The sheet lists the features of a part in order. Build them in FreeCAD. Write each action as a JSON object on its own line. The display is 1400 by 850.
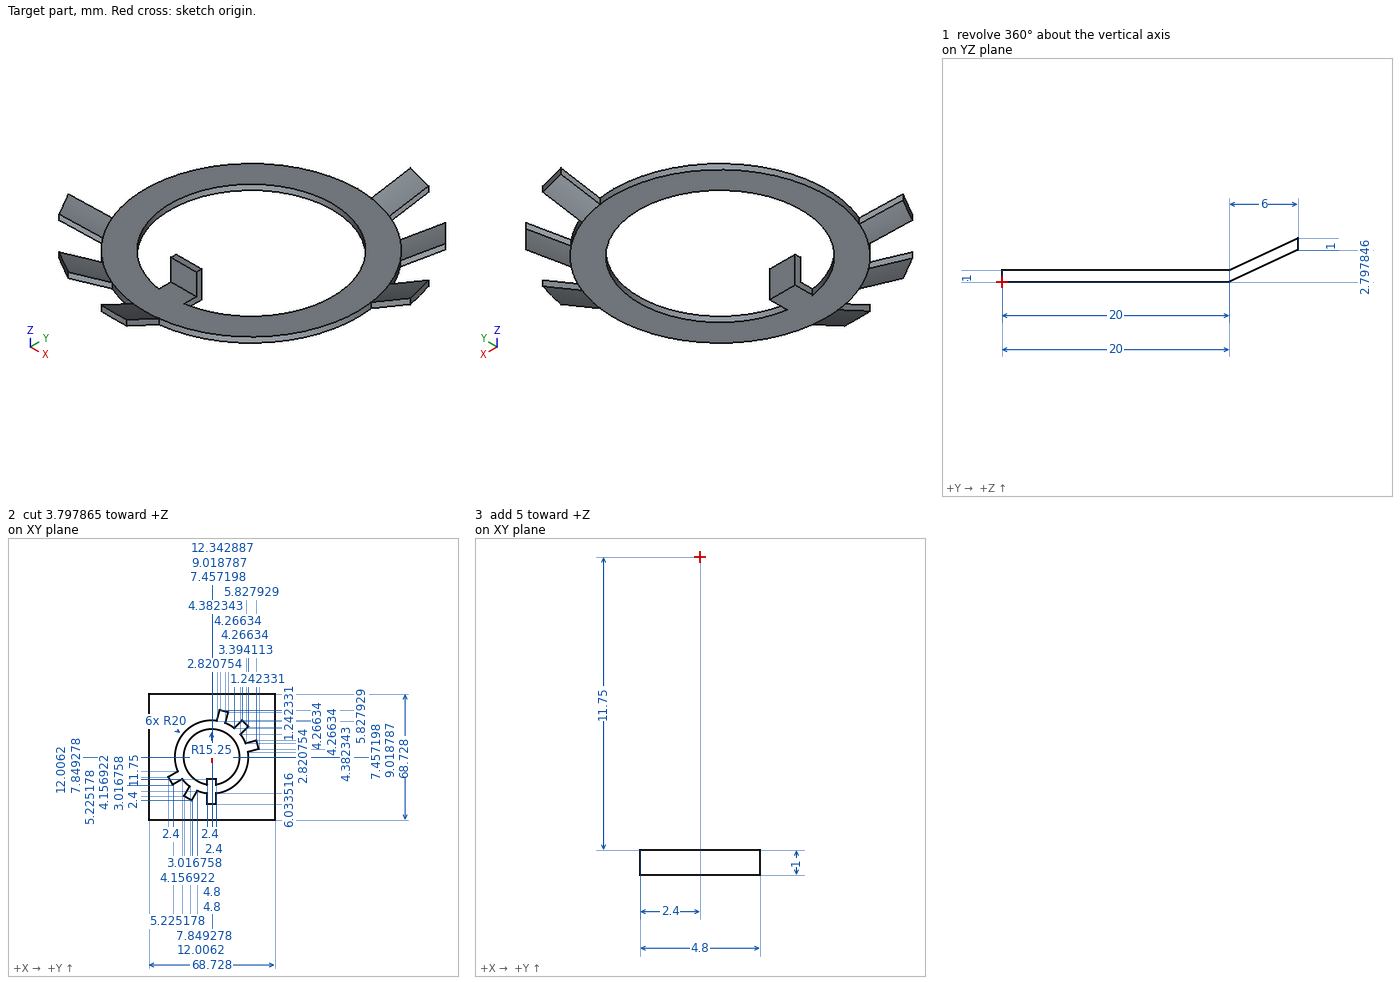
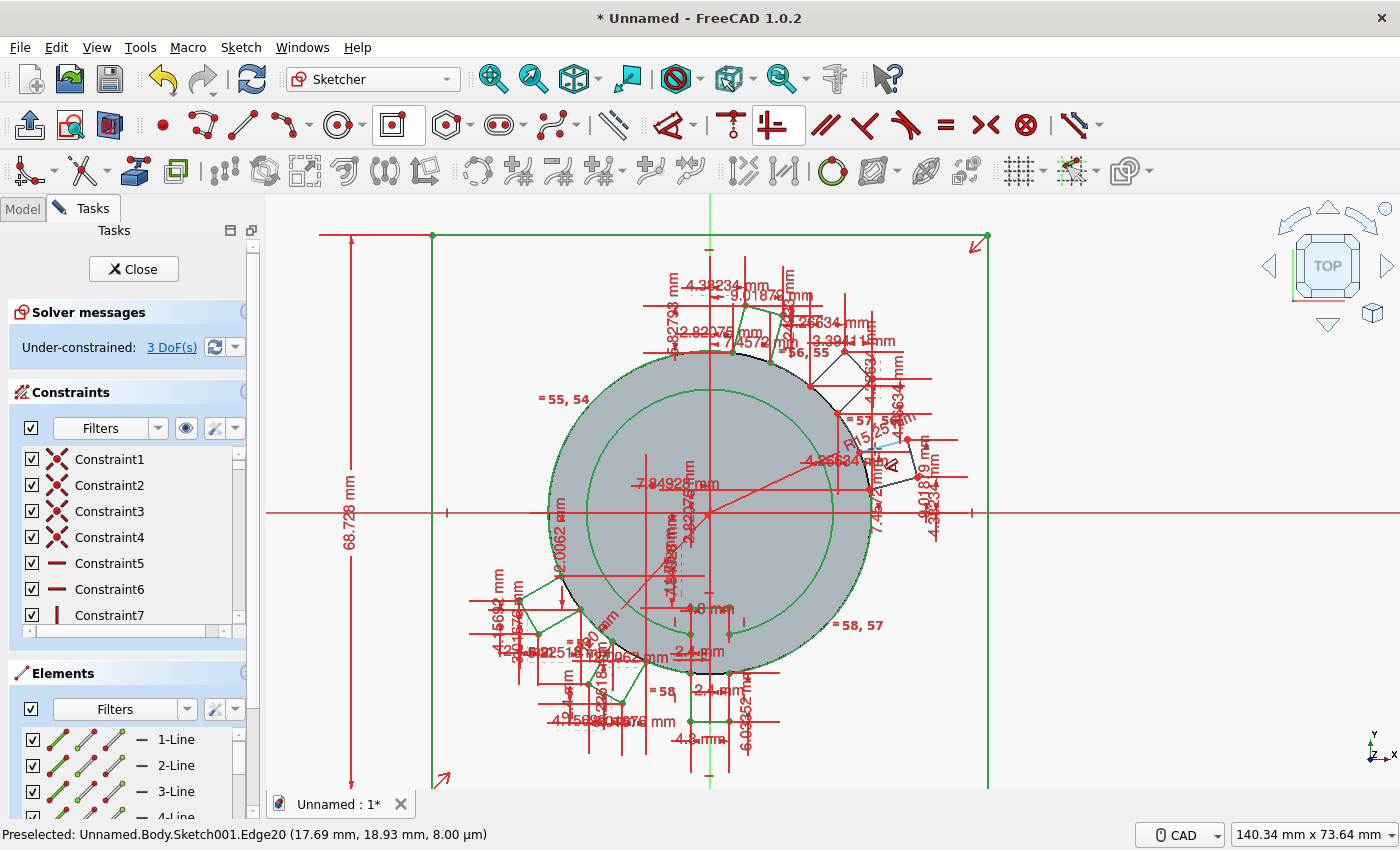
{"action": "left_click", "coordinate": [874, 449]}
{"action": "left_click", "coordinate": [884, 534]}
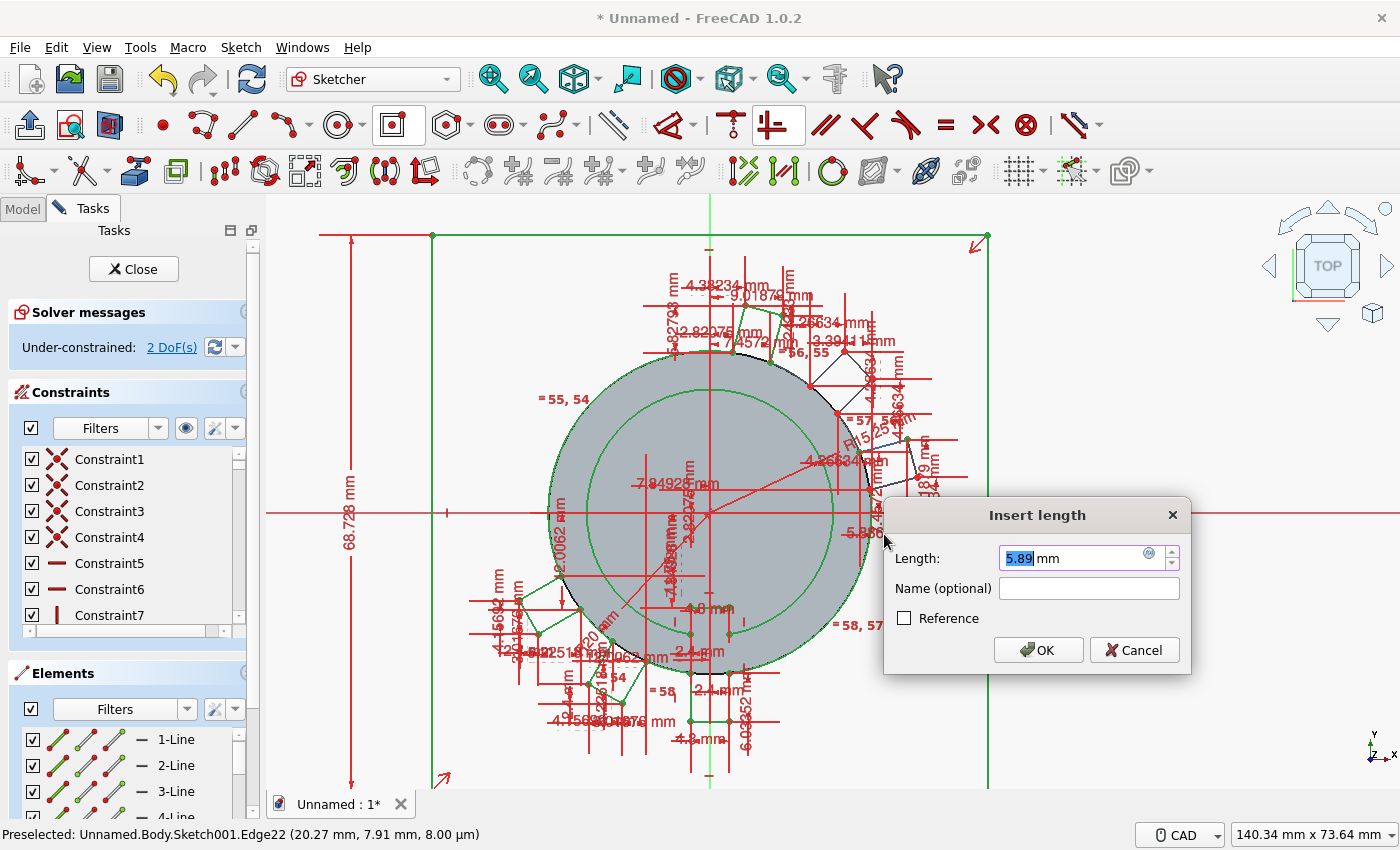
{"action": "type", "text": "5.827929"}
{"action": "key", "text": "Return"}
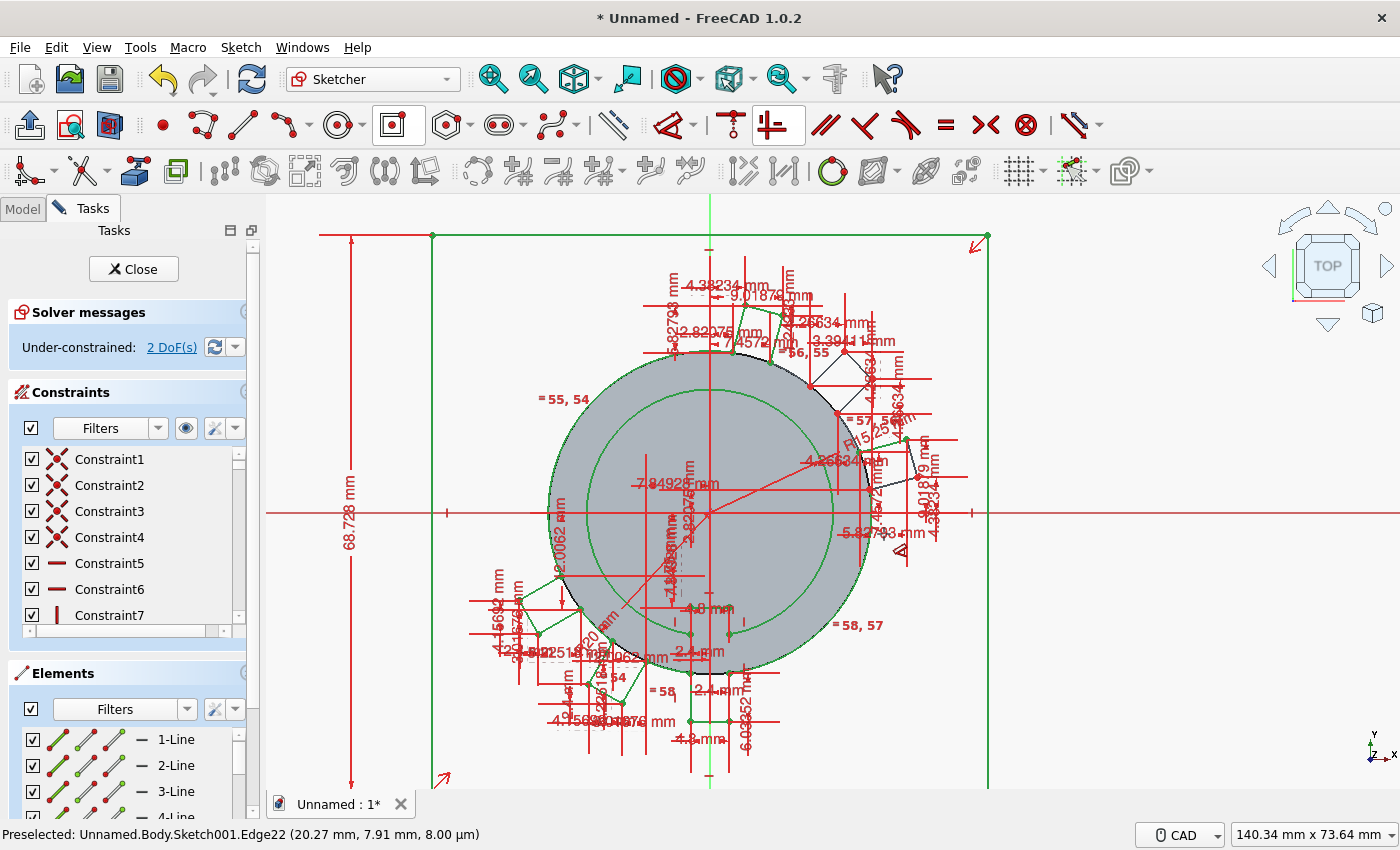
{"action": "scroll", "coordinate": [910, 451], "scroll_direction": "up", "scroll_amount": 7}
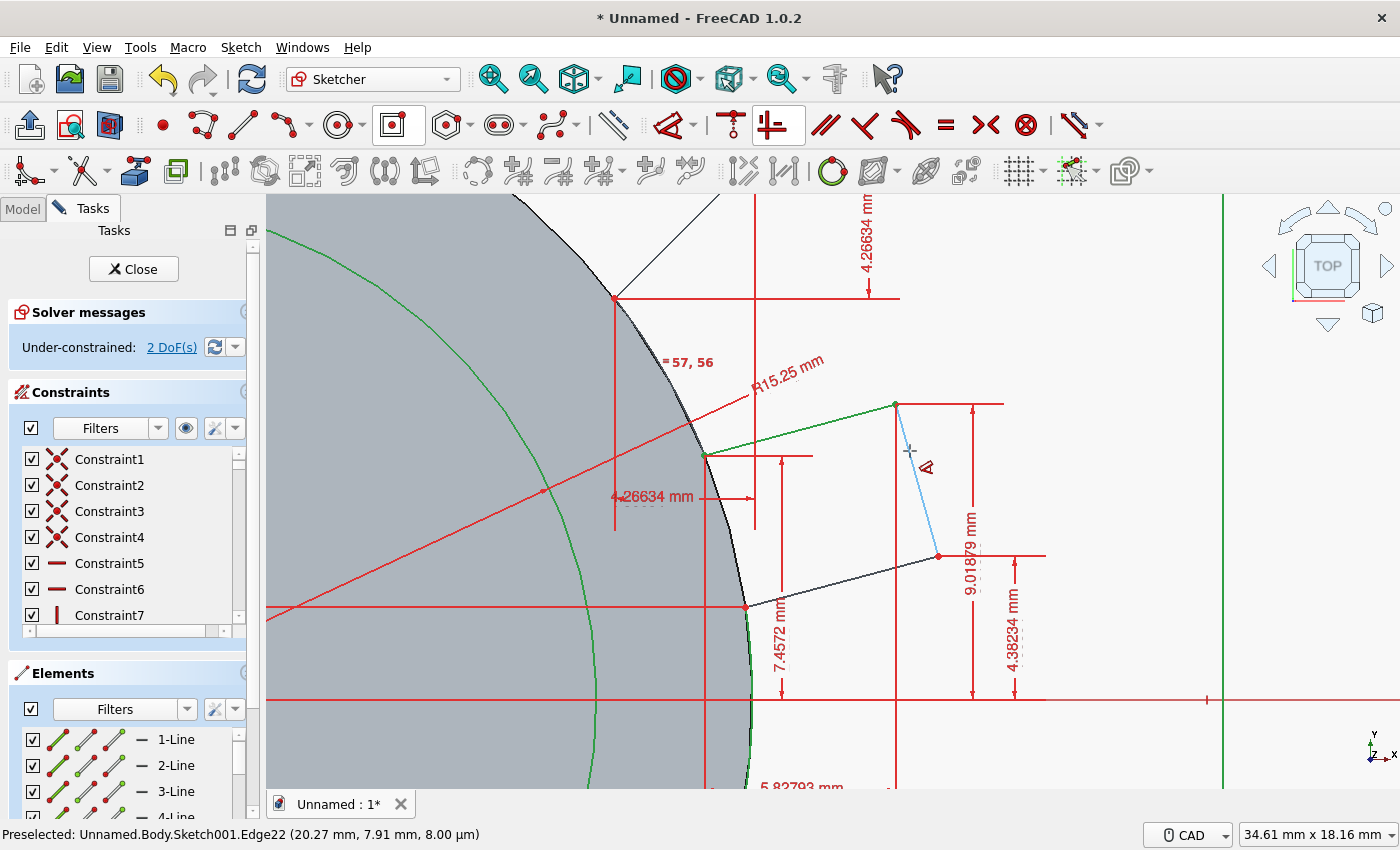
{"action": "left_click", "coordinate": [909, 450]}
{"action": "left_click", "coordinate": [917, 370]}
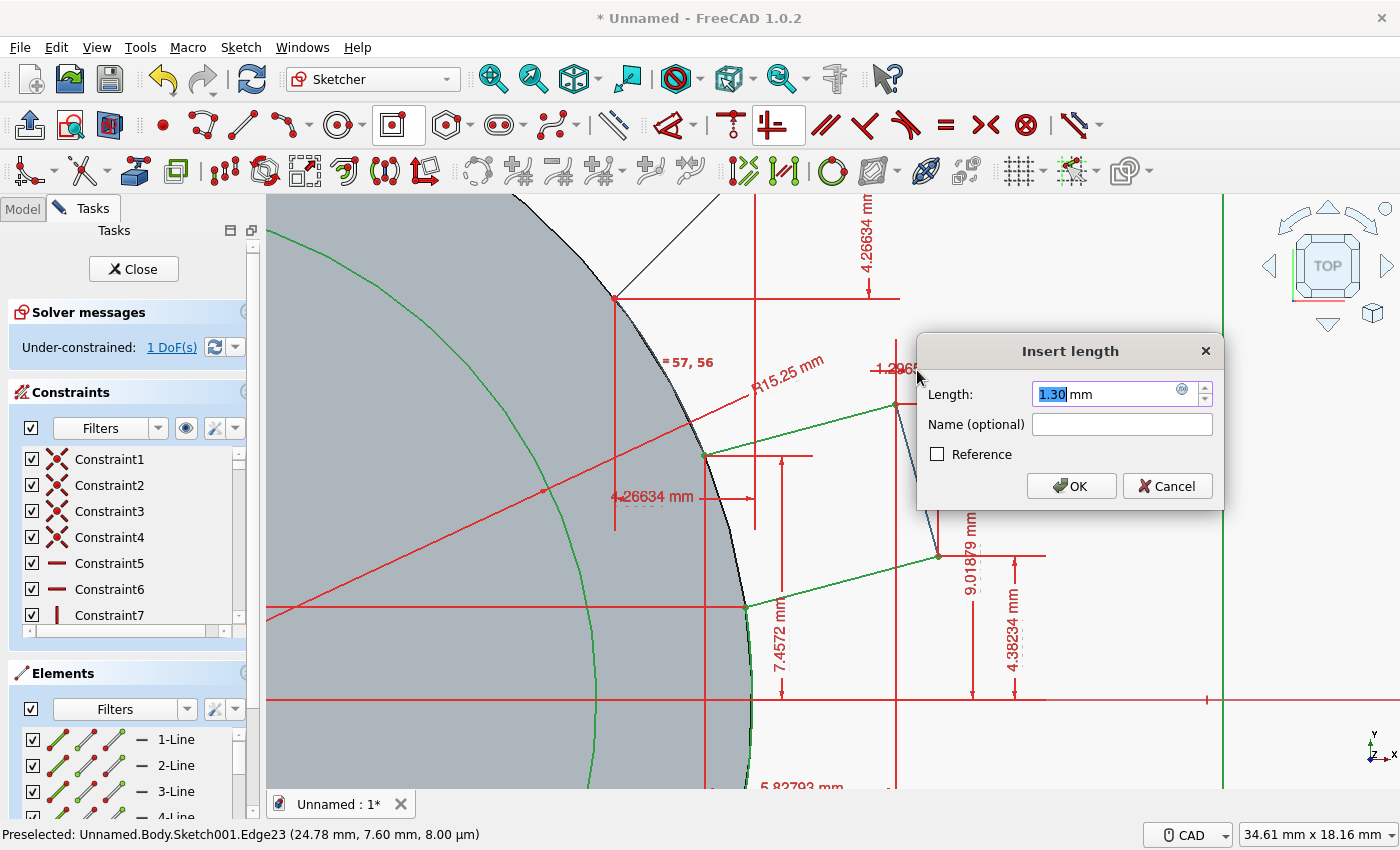
{"action": "type", "text": "1.242331"}
{"action": "key", "text": "Return"}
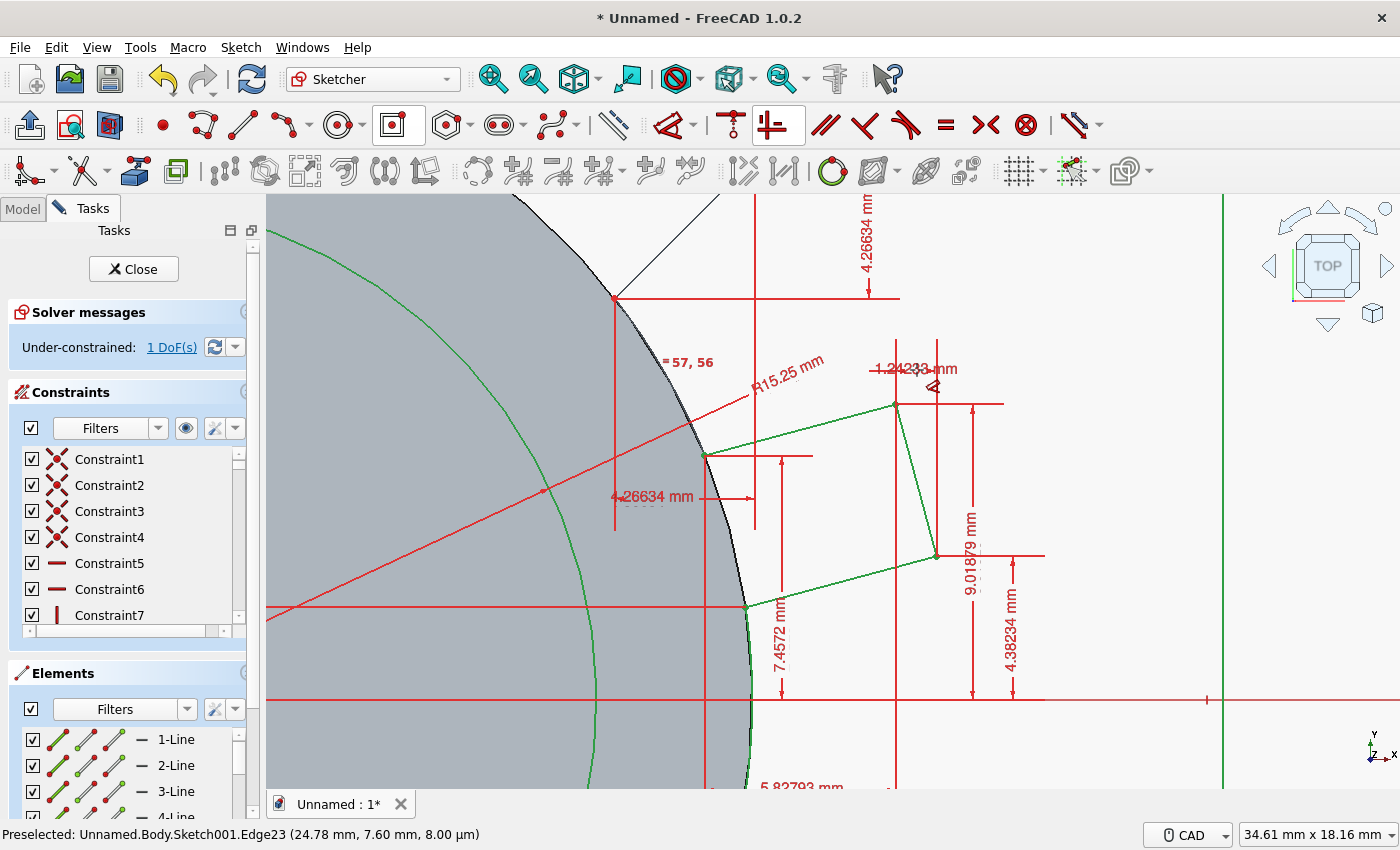
{"action": "scroll", "coordinate": [897, 450], "scroll_direction": "down", "scroll_amount": 9}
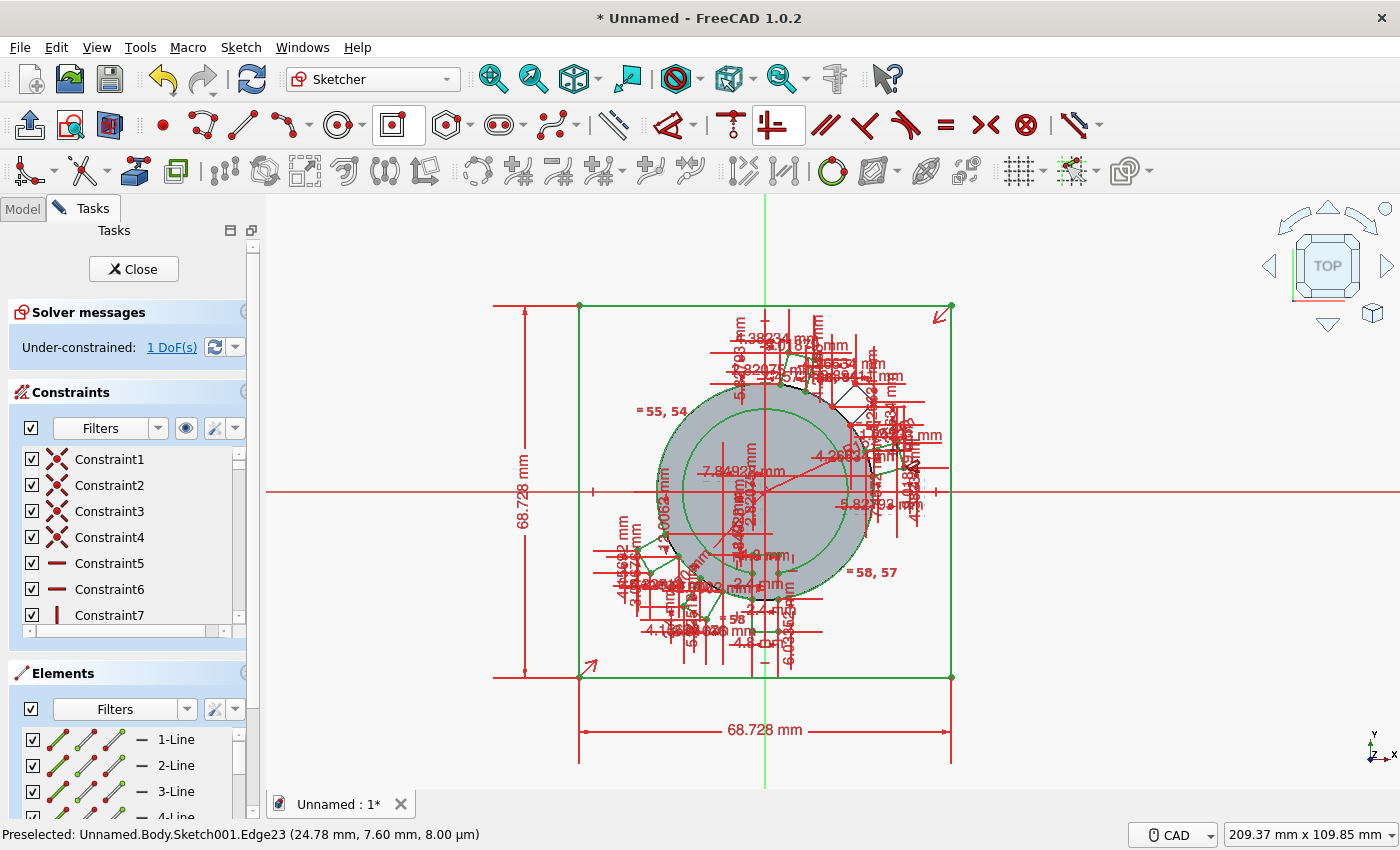
{"action": "left_click", "coordinate": [832, 407]}
{"action": "left_click", "coordinate": [799, 277]}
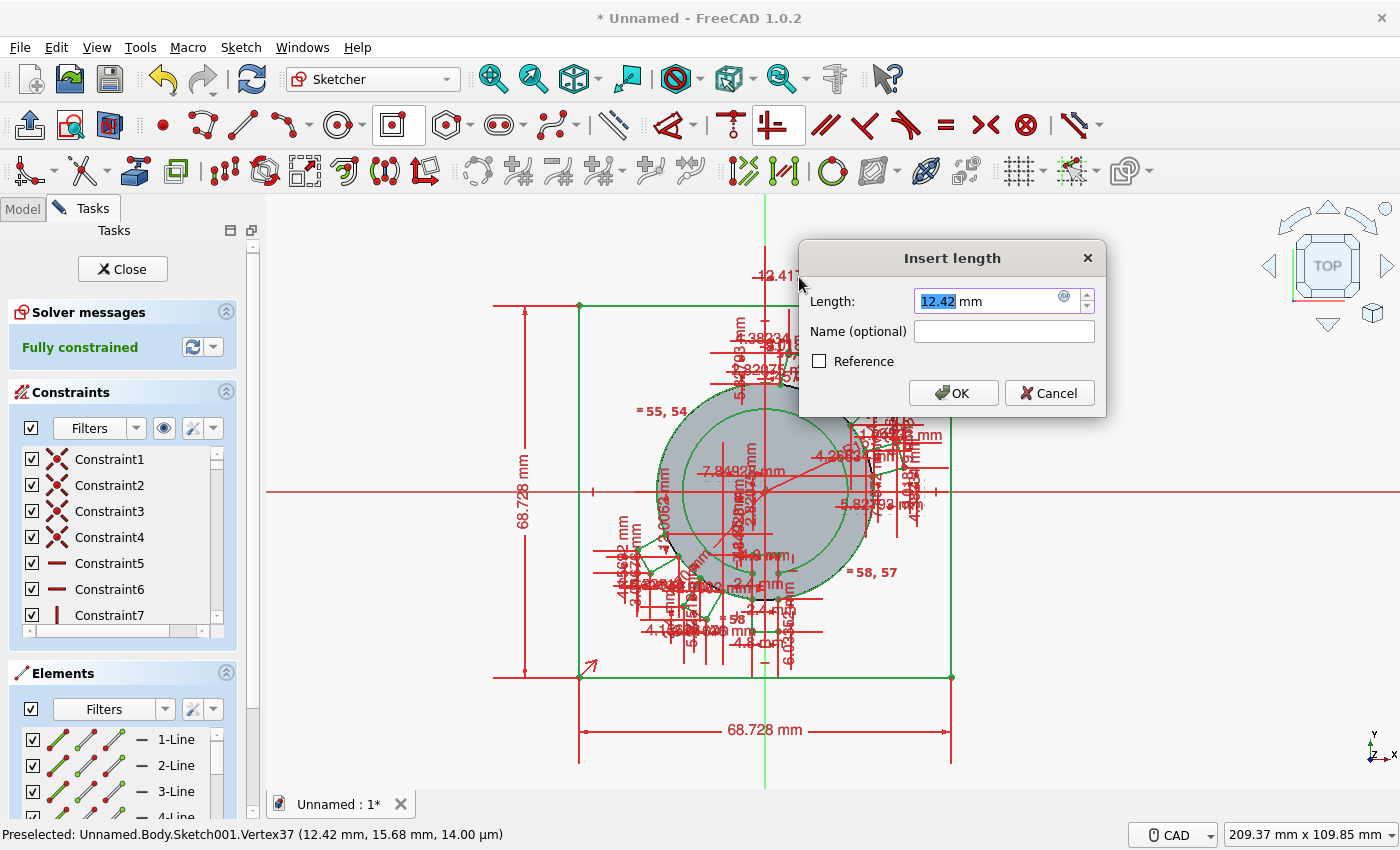
{"action": "type", "text": "12.342887"}
{"action": "key", "text": "Return"}
{"action": "key", "text": "Escape"}